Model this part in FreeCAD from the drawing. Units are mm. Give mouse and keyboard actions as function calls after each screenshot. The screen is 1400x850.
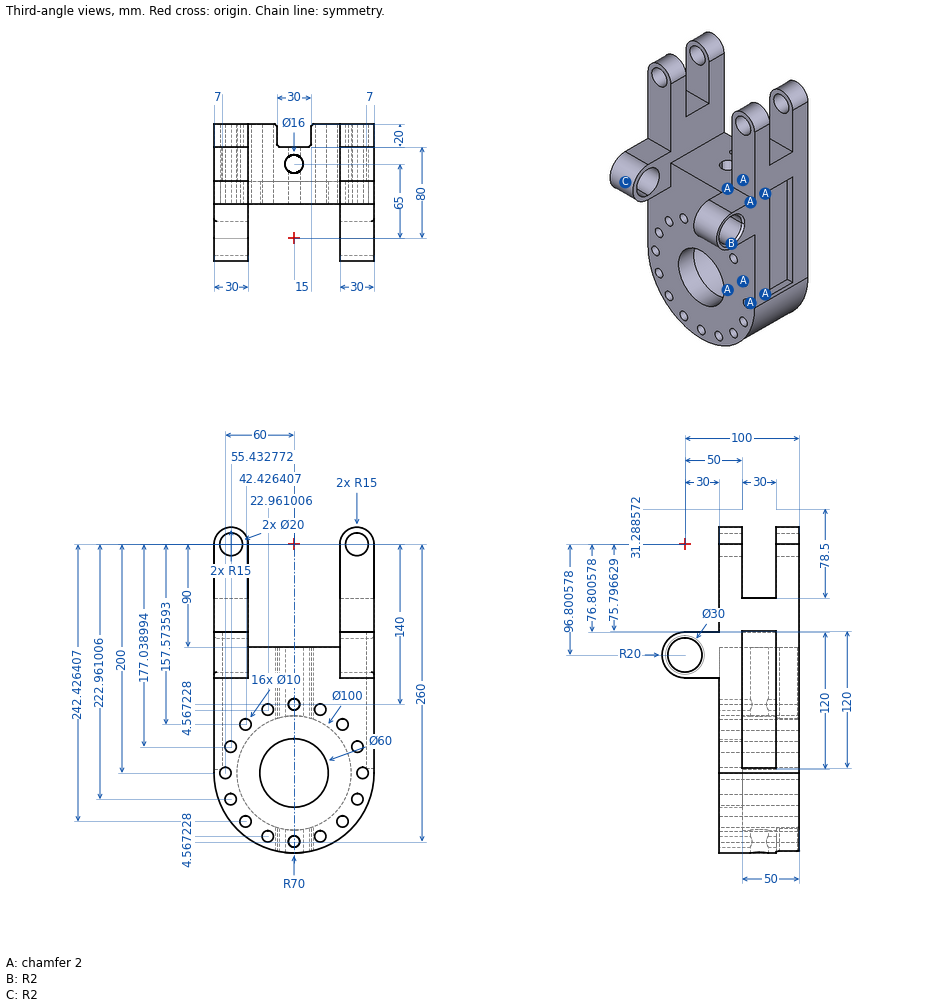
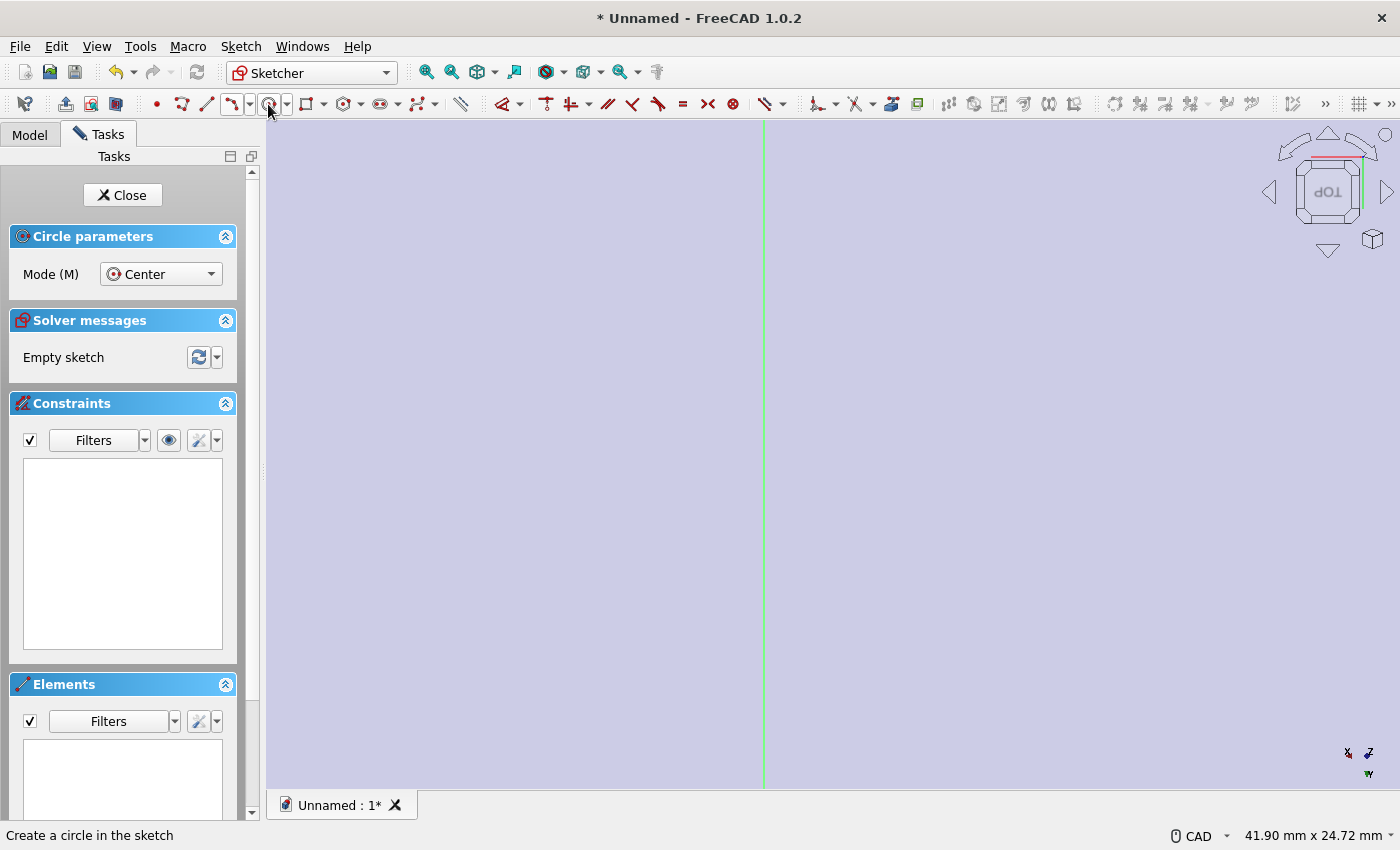
click(764, 454)
click(917, 301)
key(Escape)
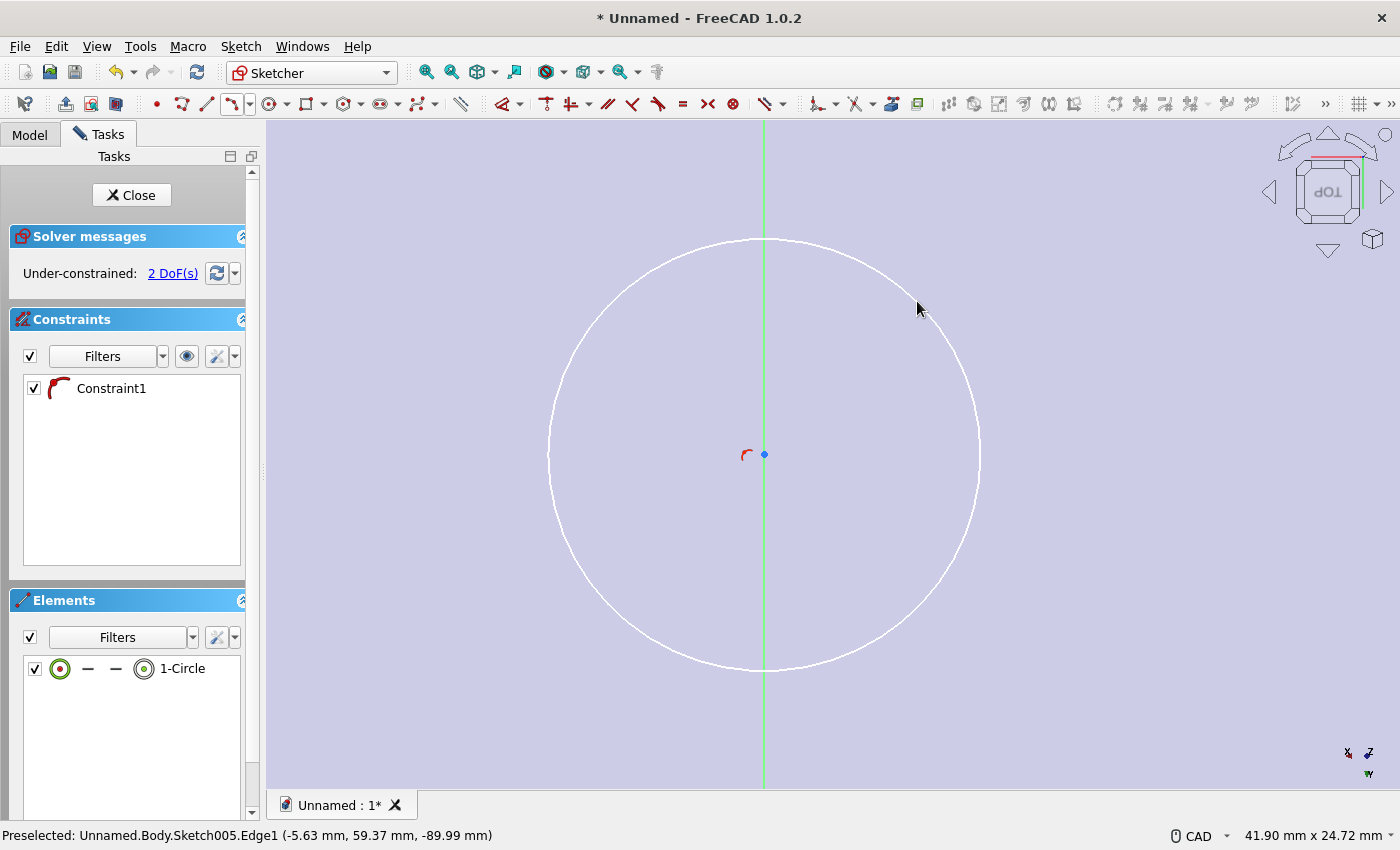
click(502, 104)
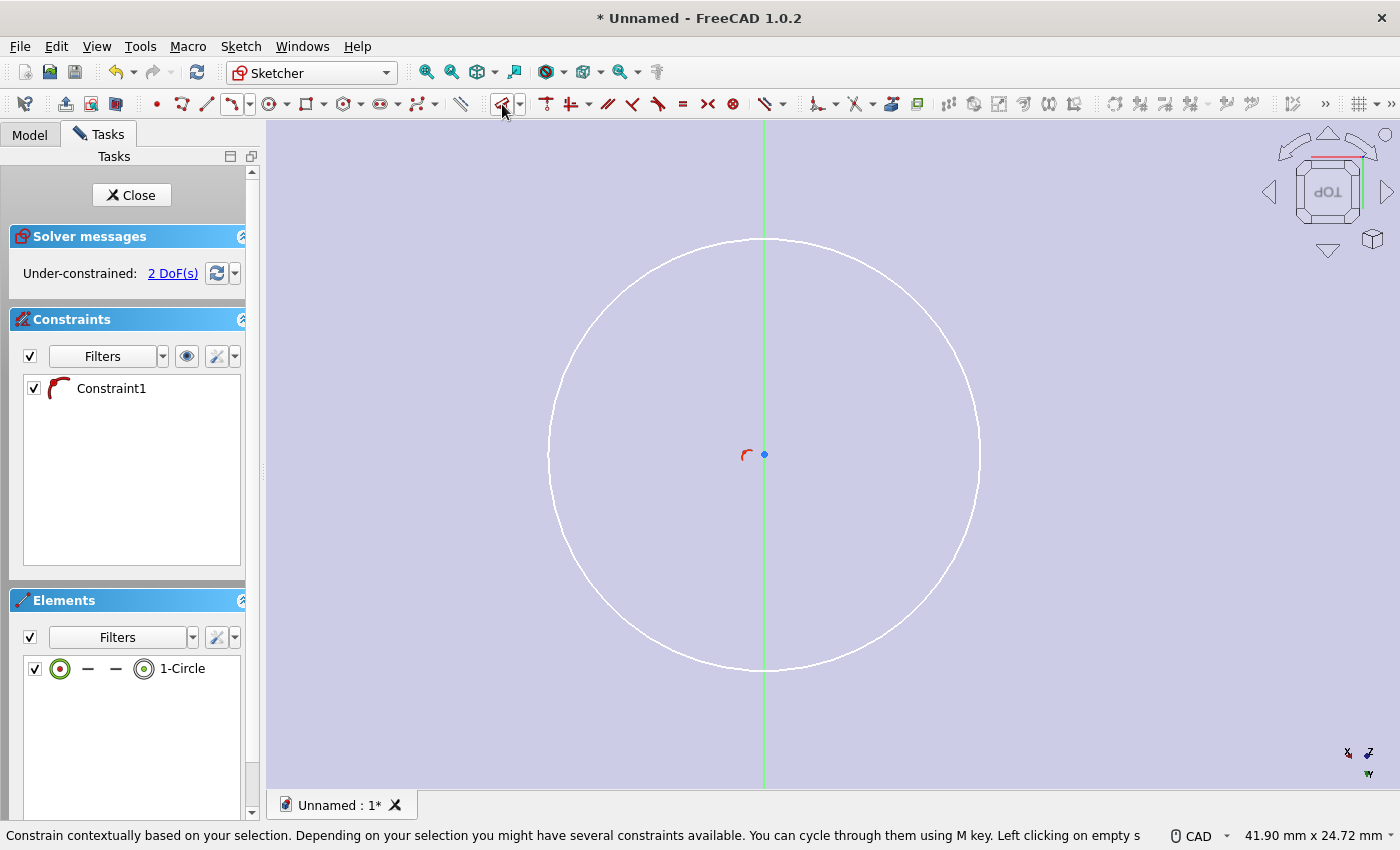
click(917, 302)
click(940, 279)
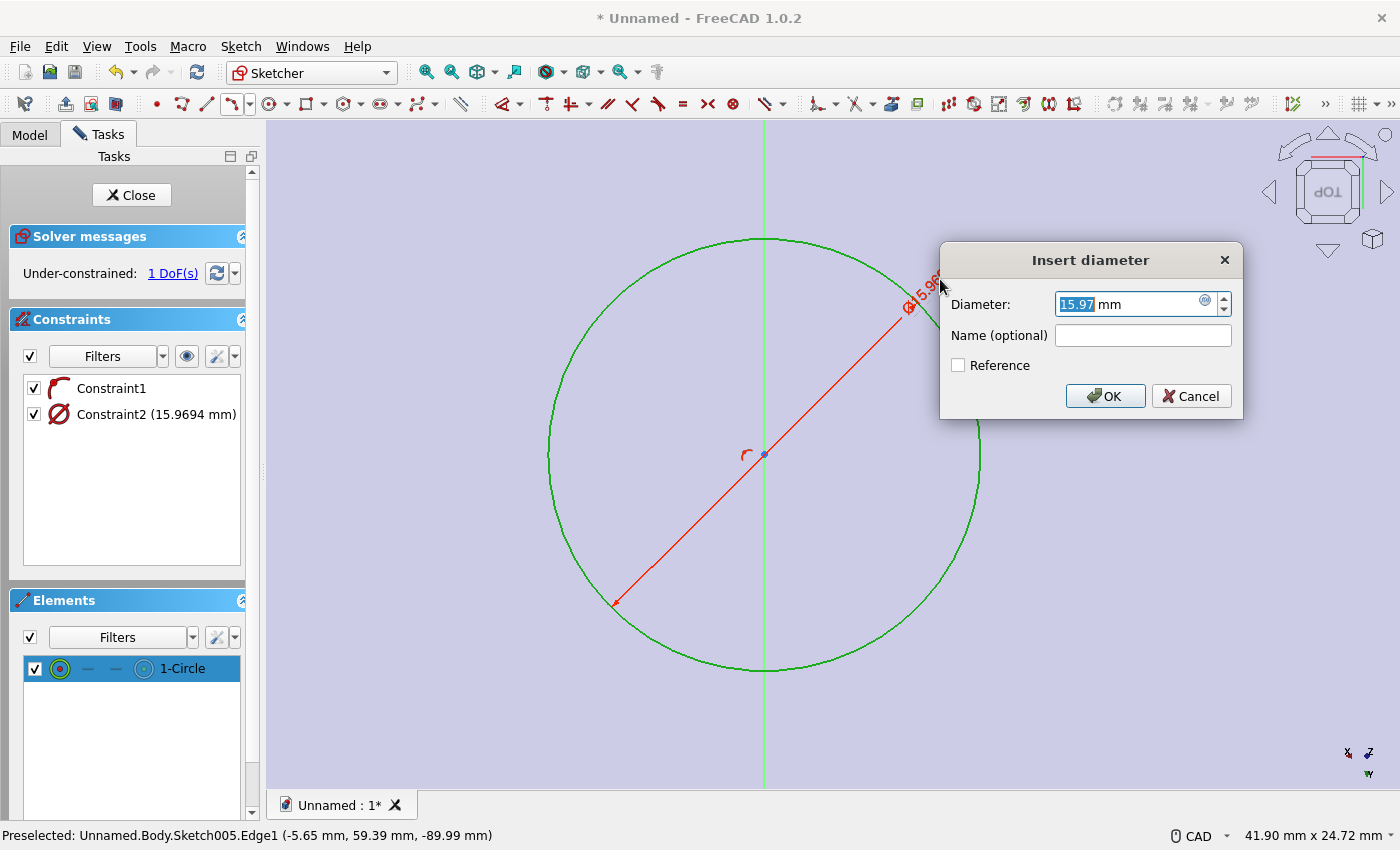
text(16)
key(Return)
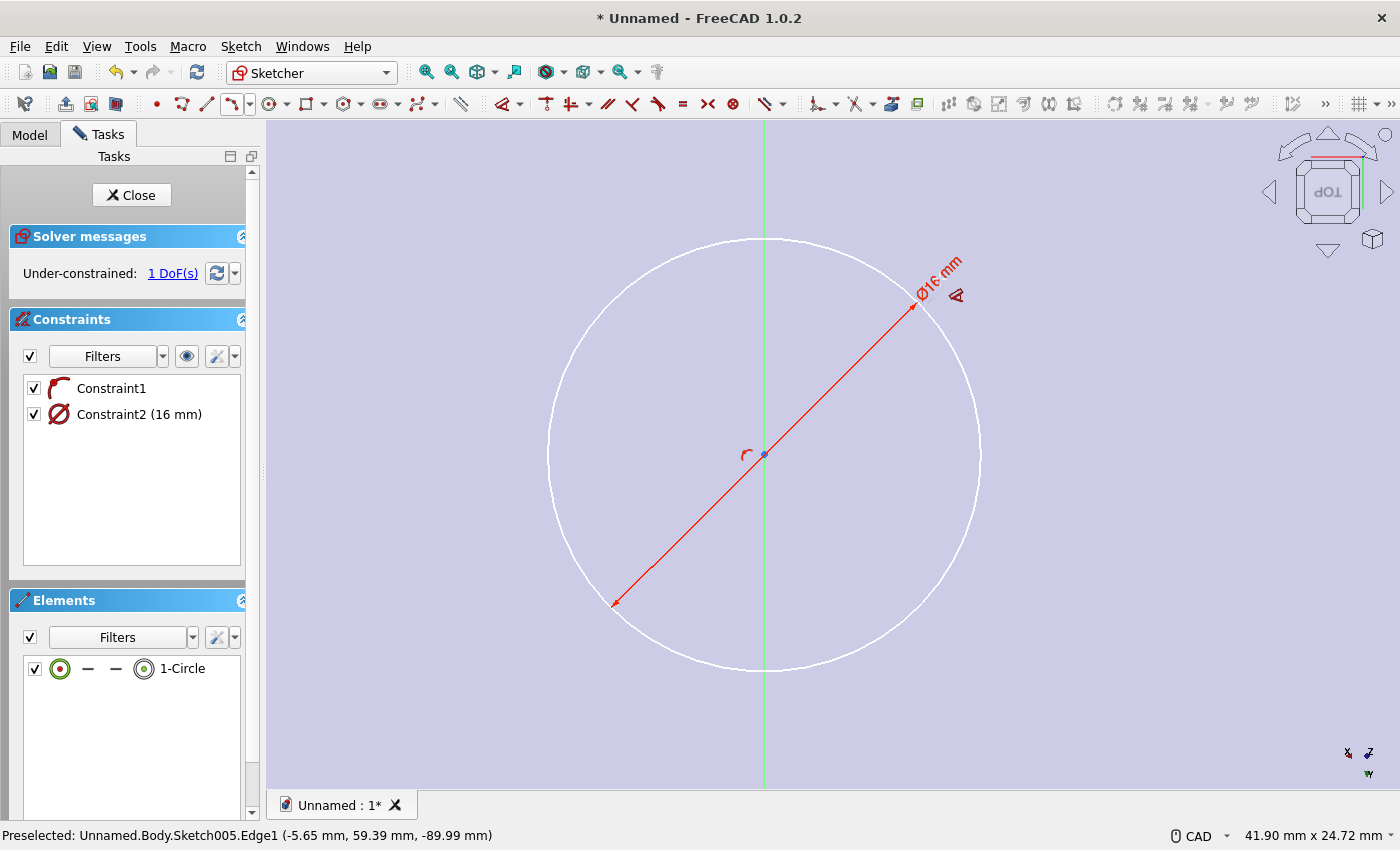
click(764, 455)
click(798, 301)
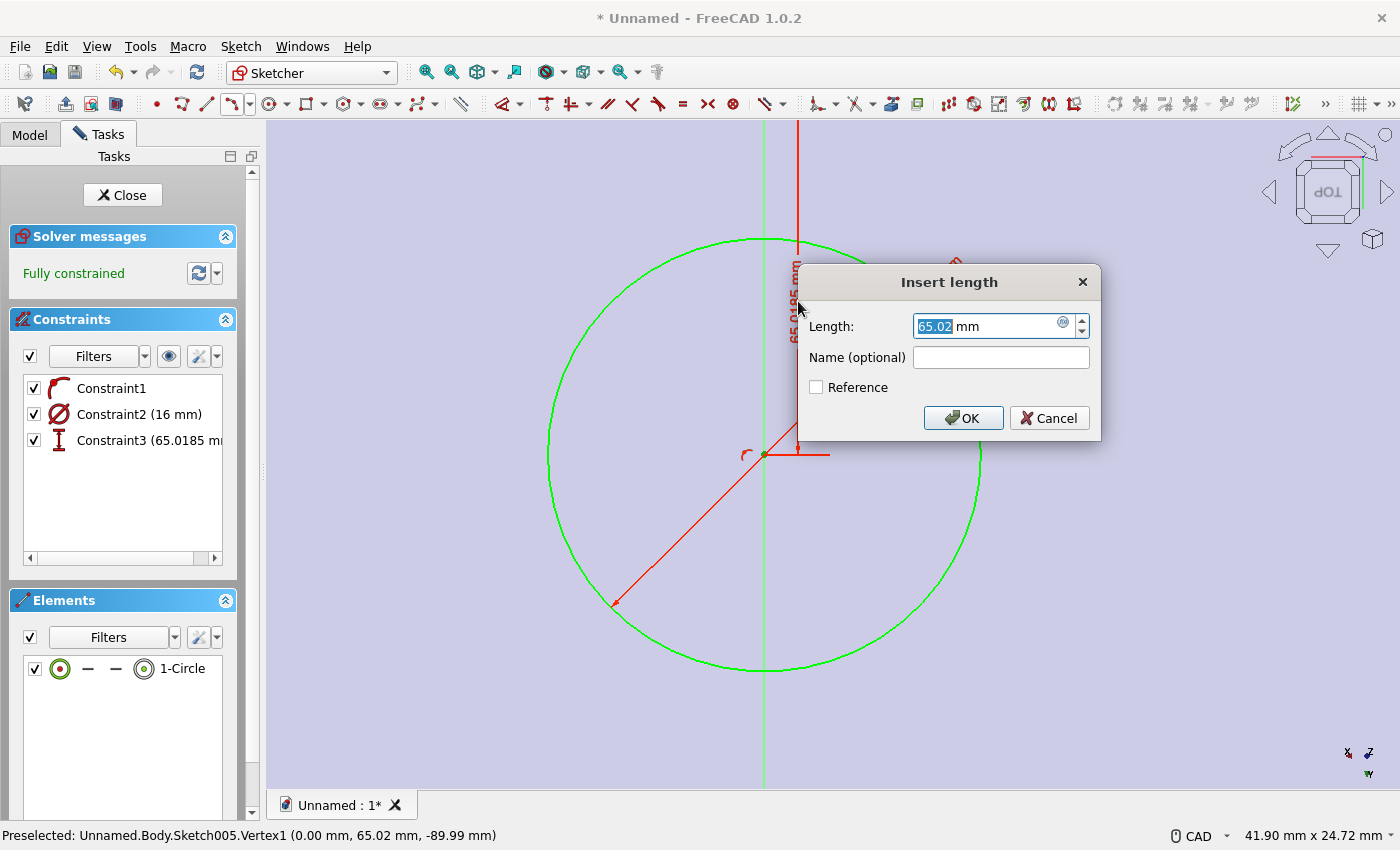
text(65)
key(Return)
key(Escape)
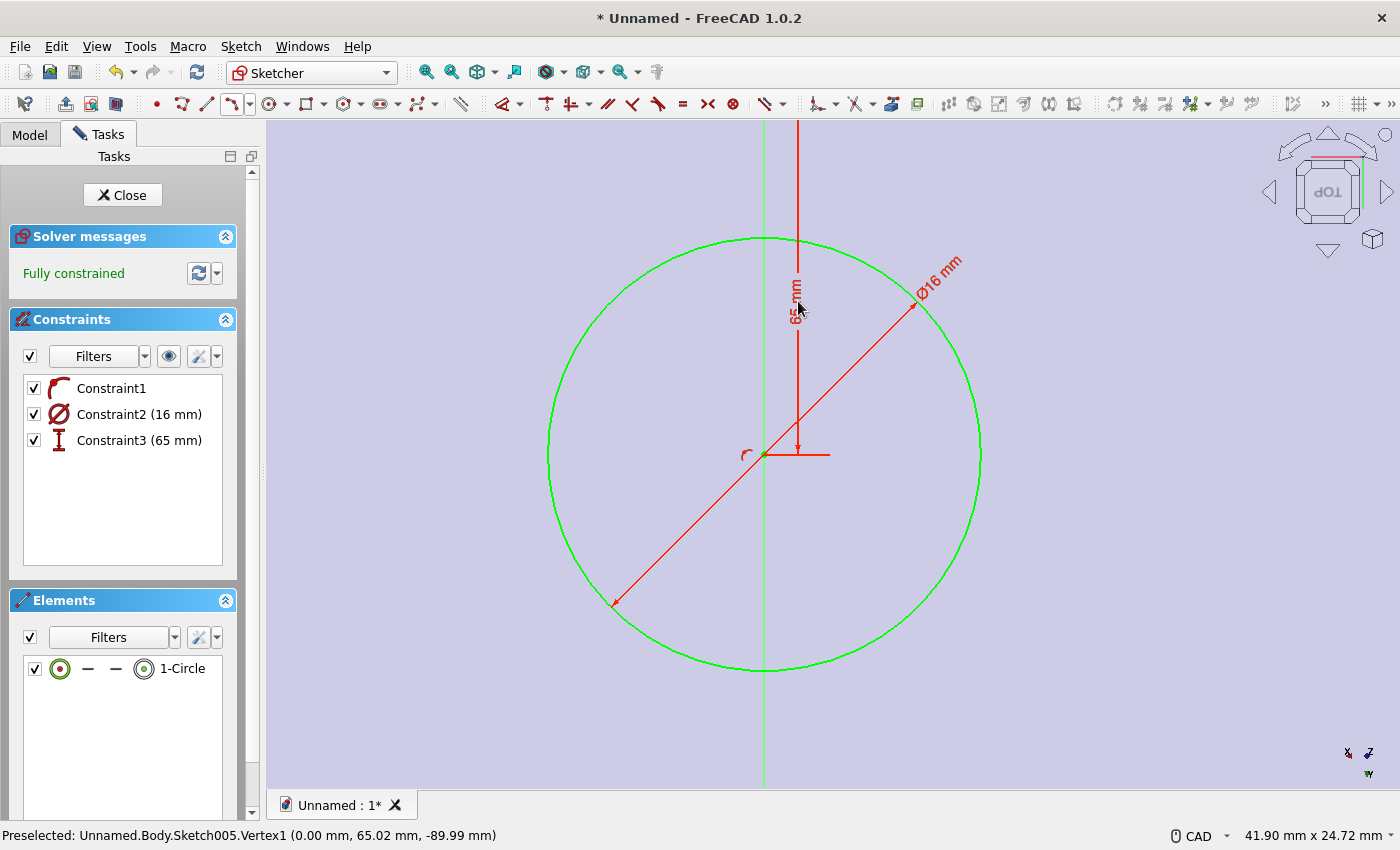
click(123, 195)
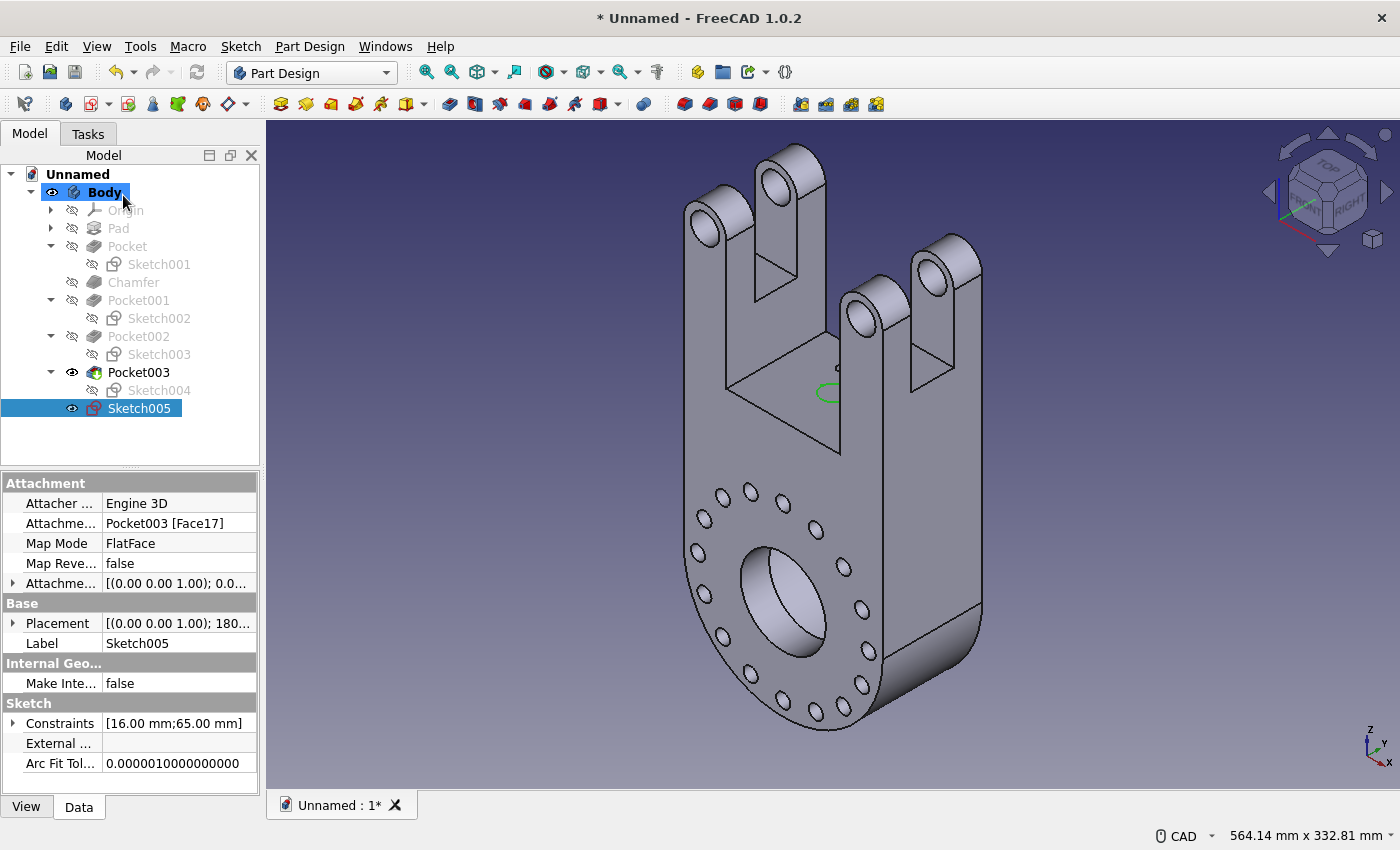
click(450, 104)